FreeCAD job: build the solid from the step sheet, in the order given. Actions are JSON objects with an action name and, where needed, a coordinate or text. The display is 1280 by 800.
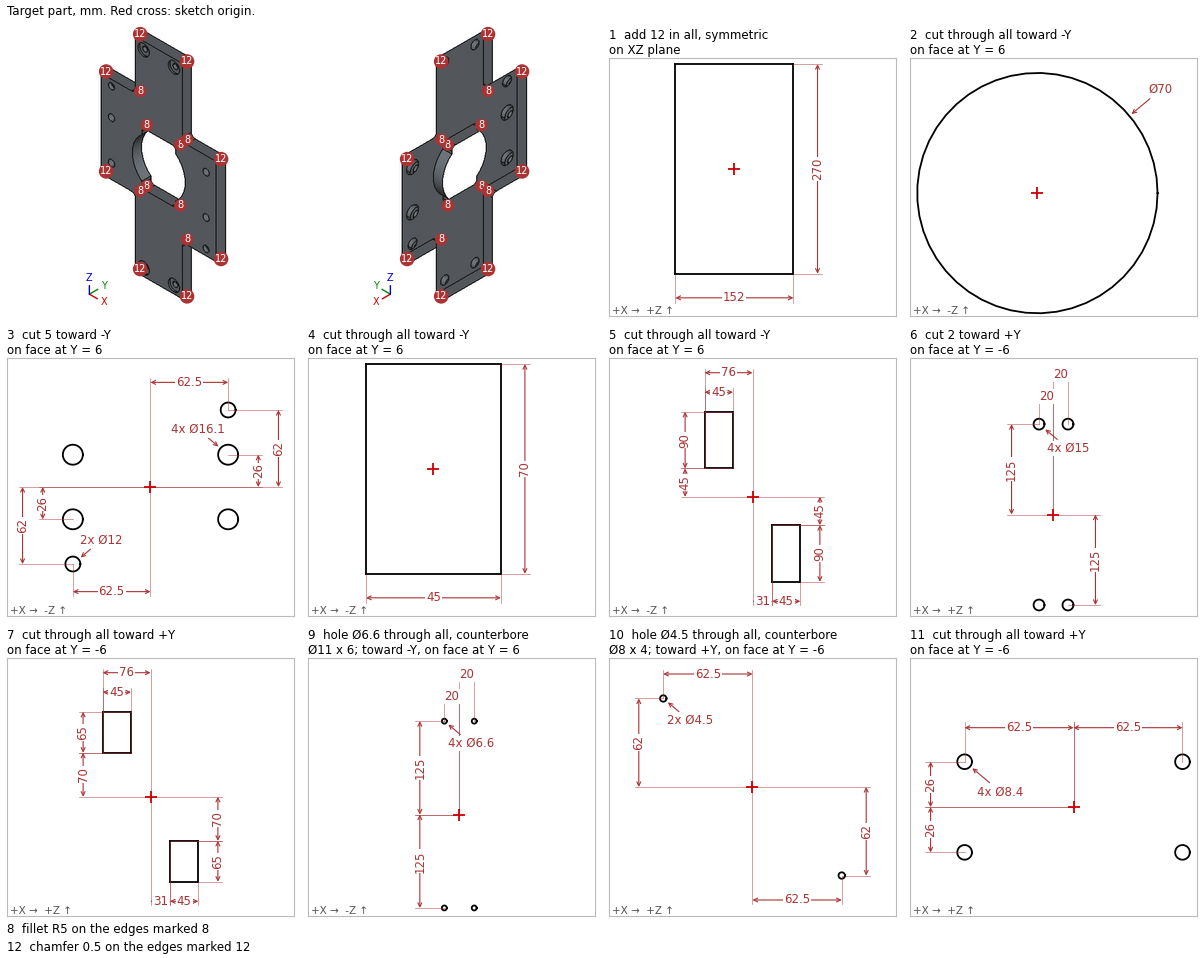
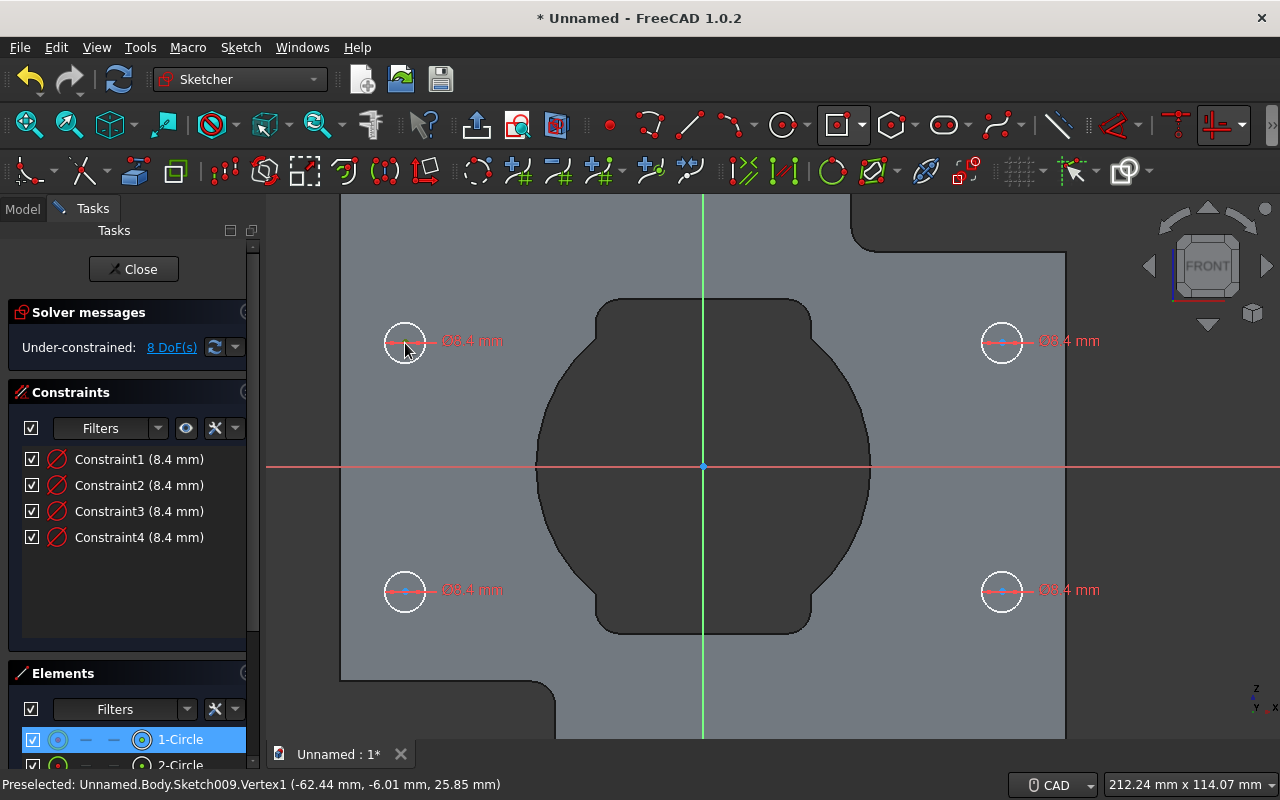
{"action": "left_click", "coordinate": [405, 592]}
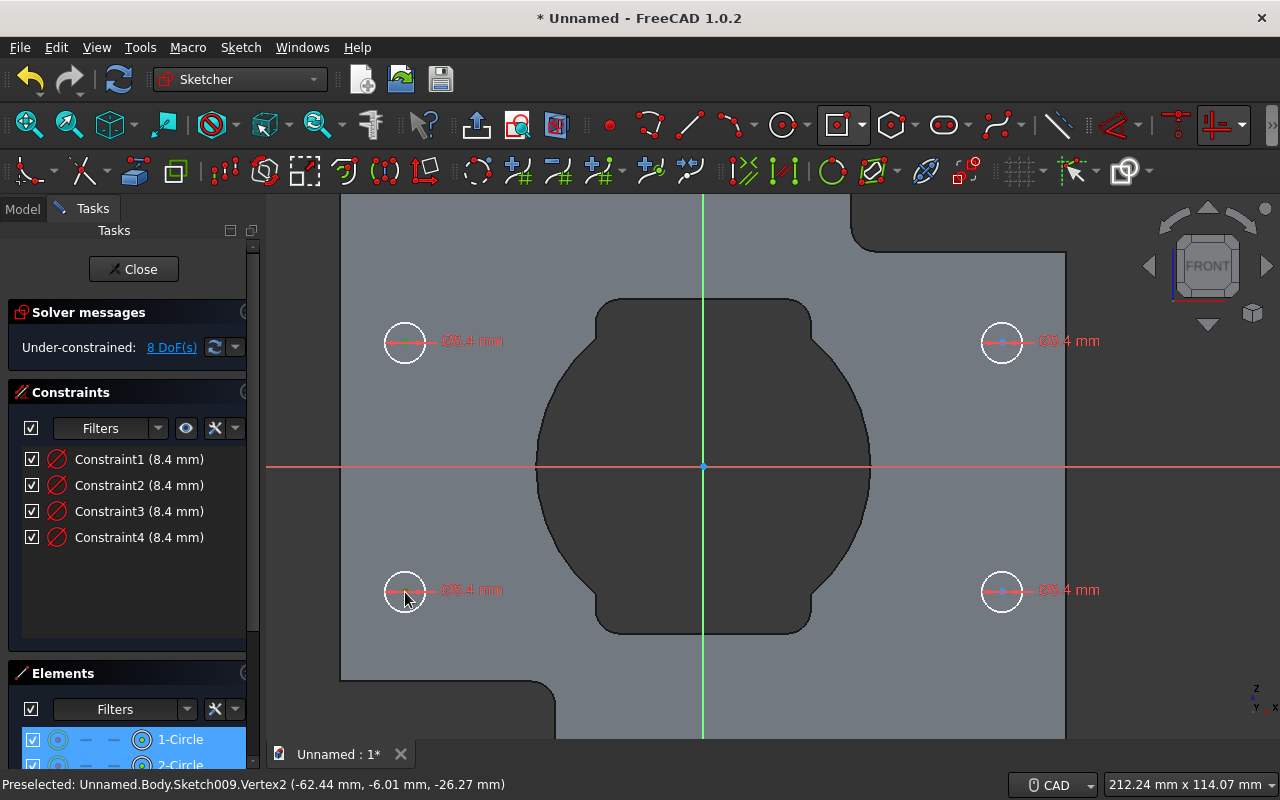
{"action": "key", "text": "v"}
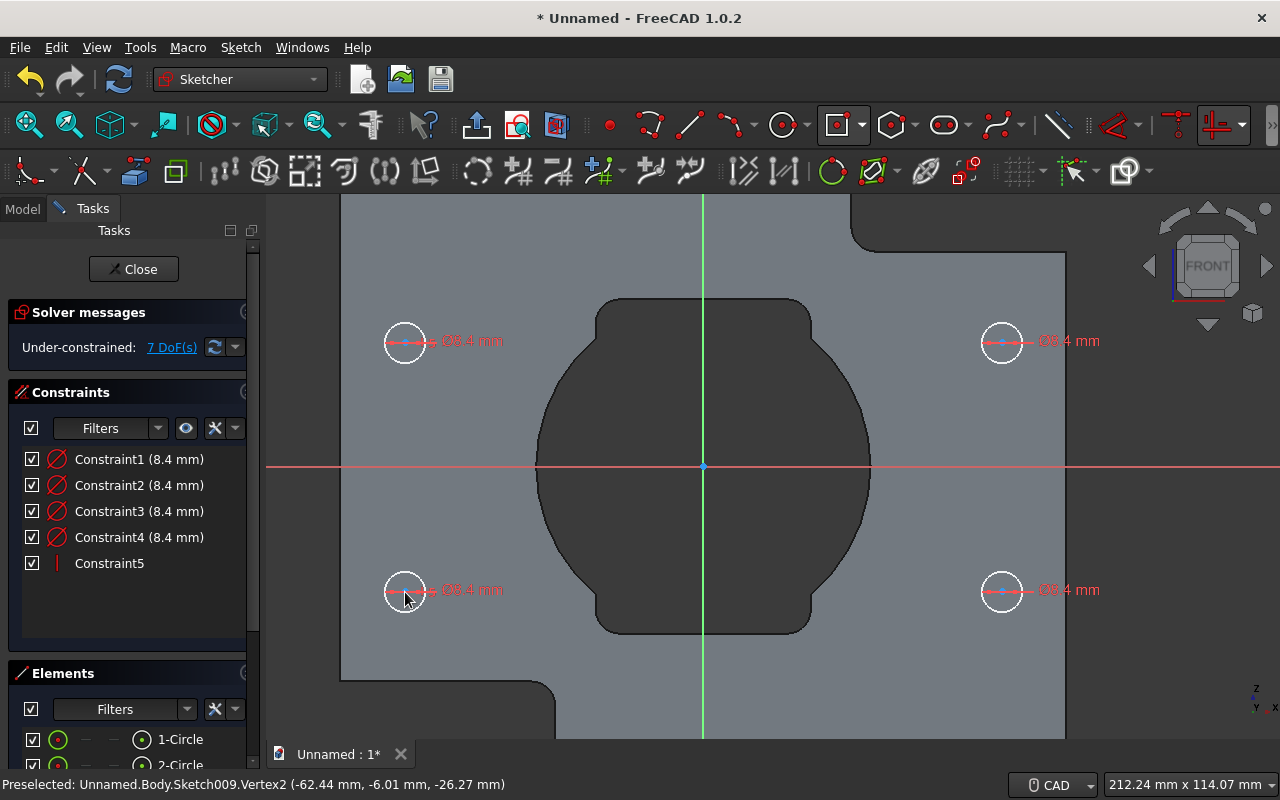
{"action": "left_click", "coordinate": [405, 343]}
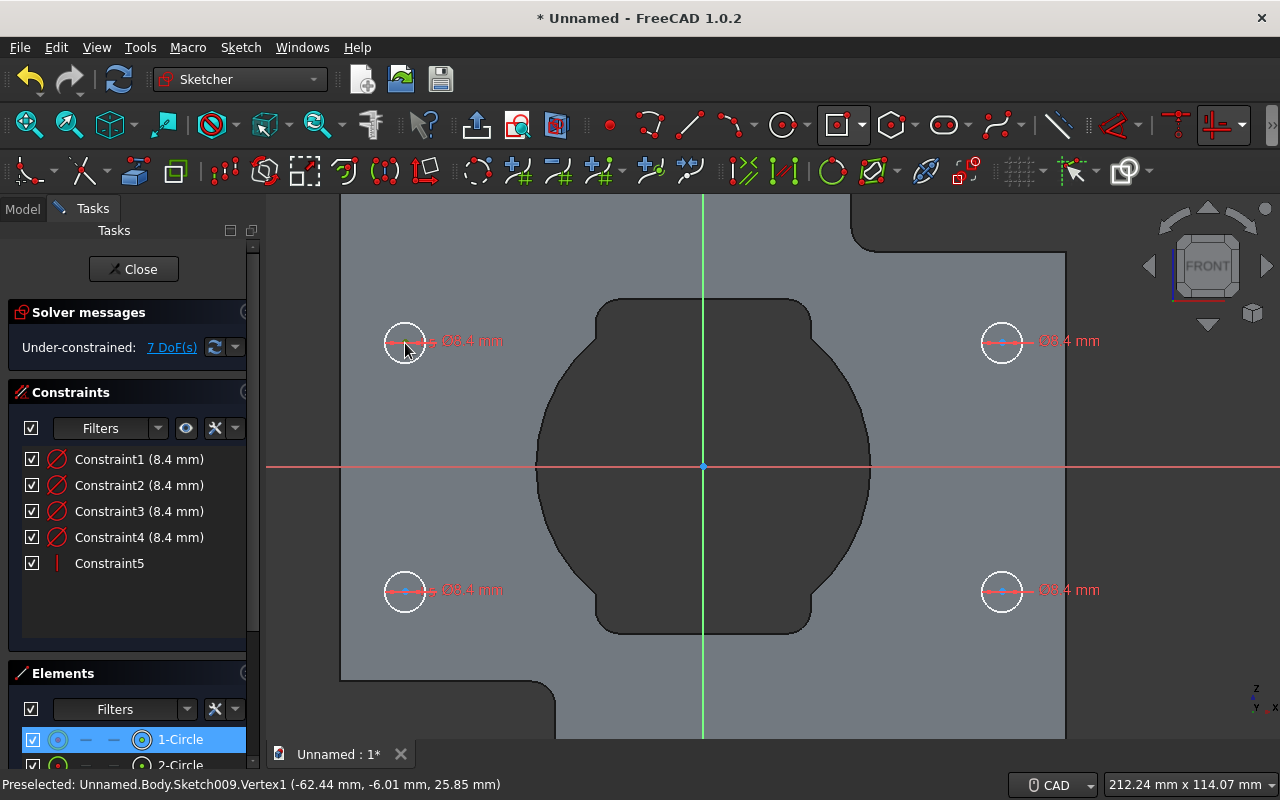
{"action": "left_click", "coordinate": [1002, 343]}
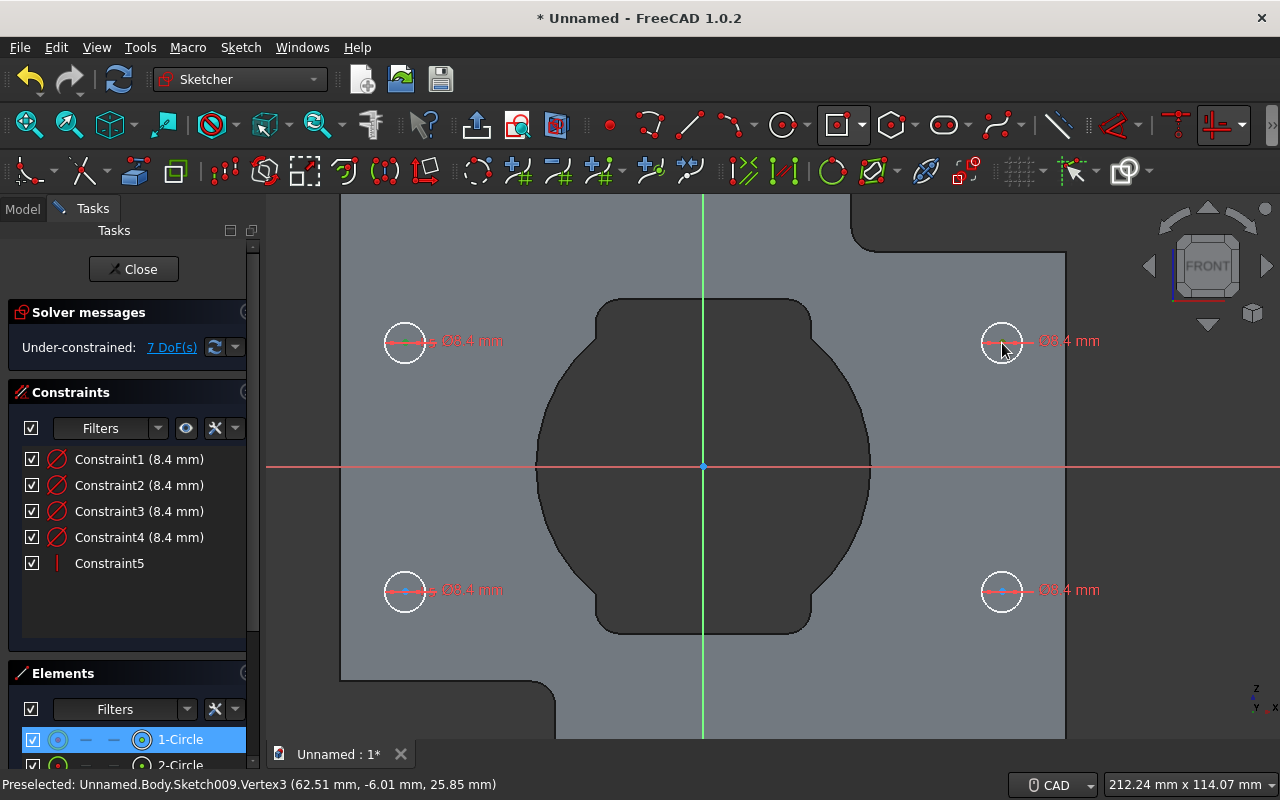
{"action": "left_click", "coordinate": [1244, 126]}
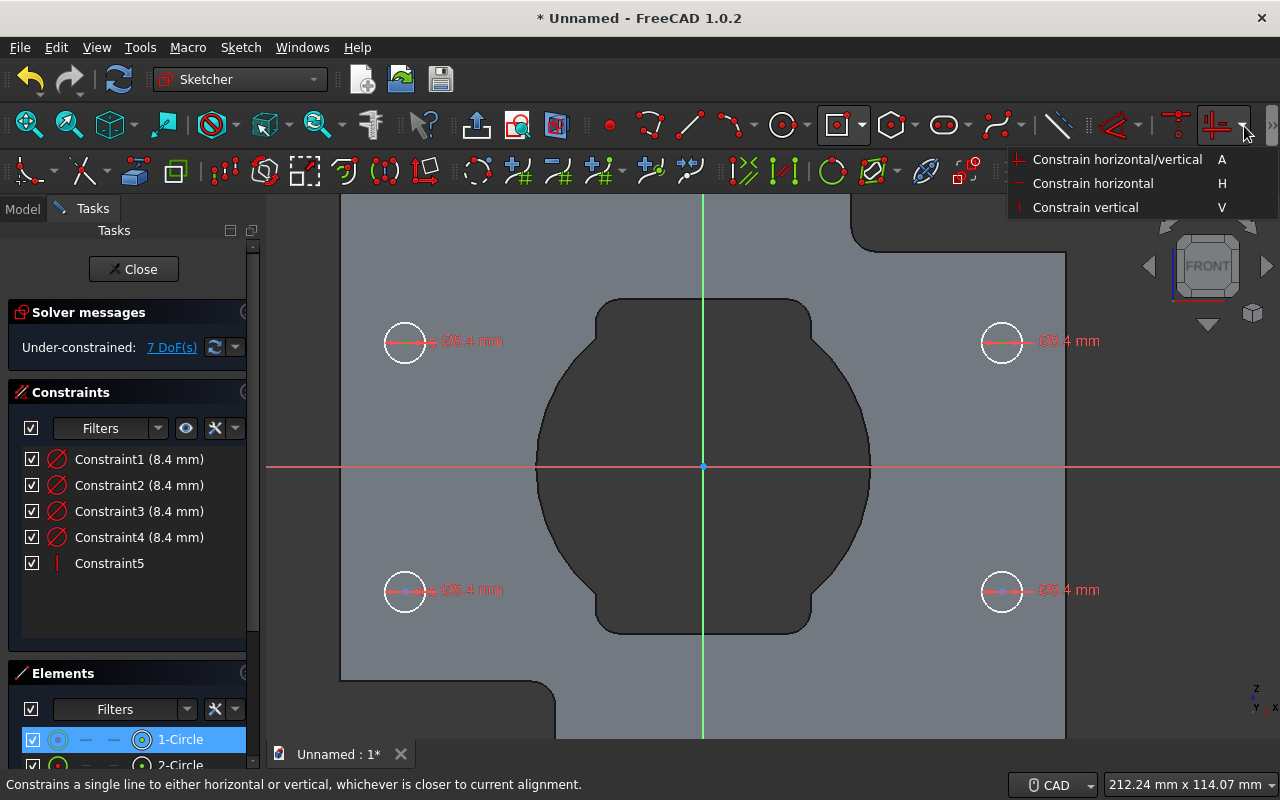
{"action": "left_click", "coordinate": [1143, 183]}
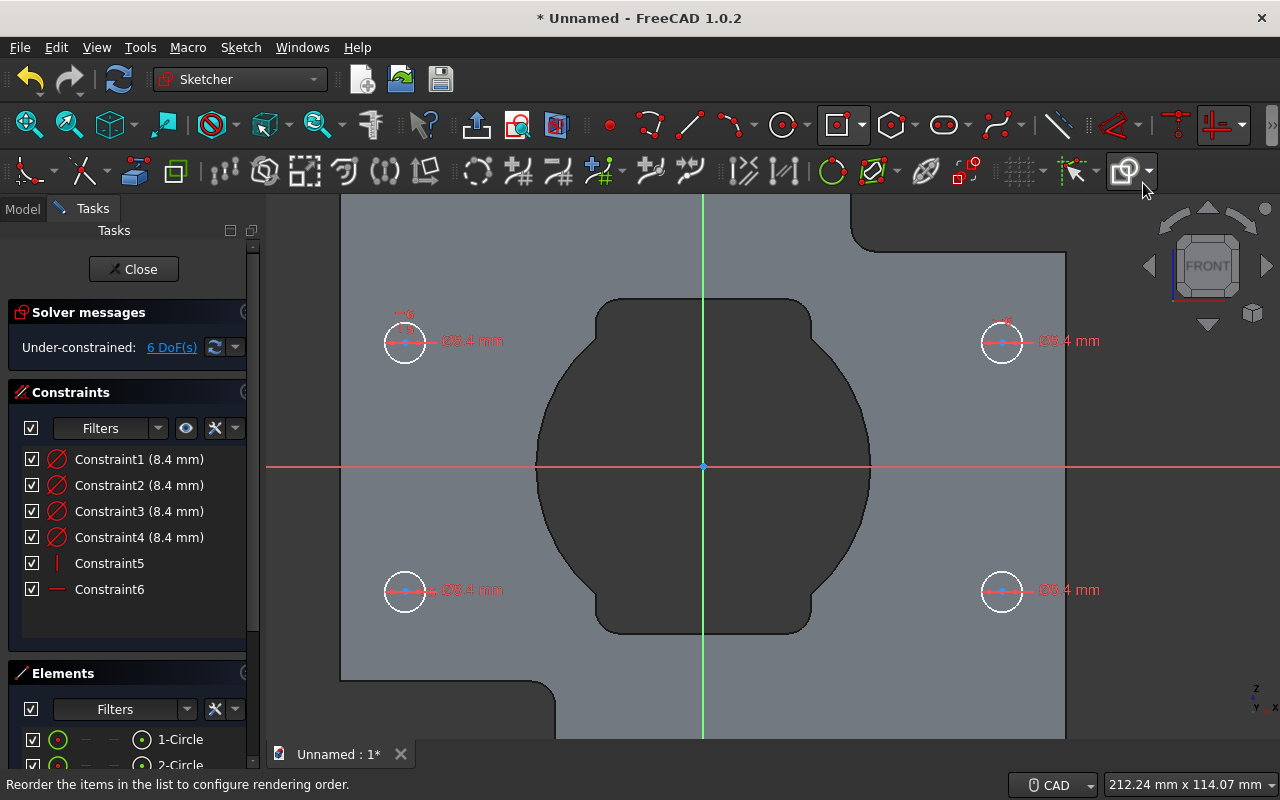
{"action": "left_click", "coordinate": [1002, 343]}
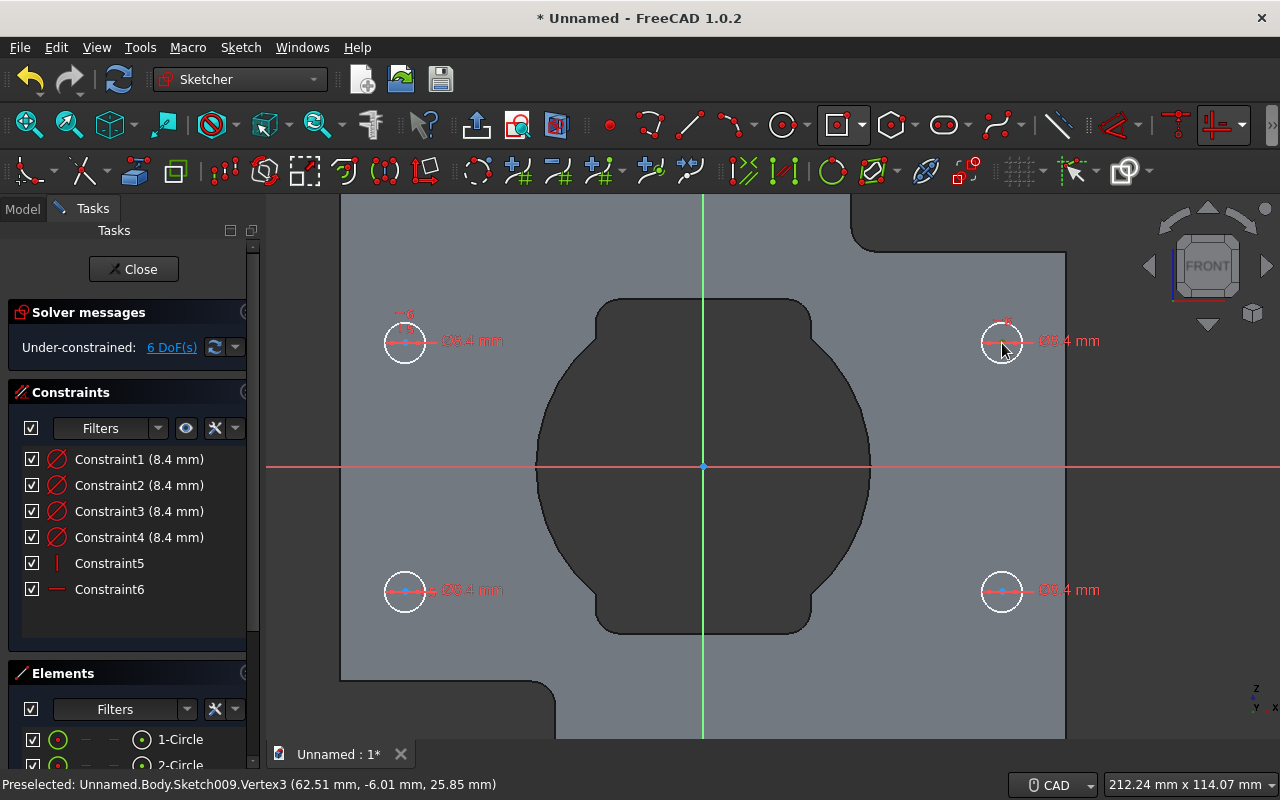
{"action": "left_click", "coordinate": [1002, 592]}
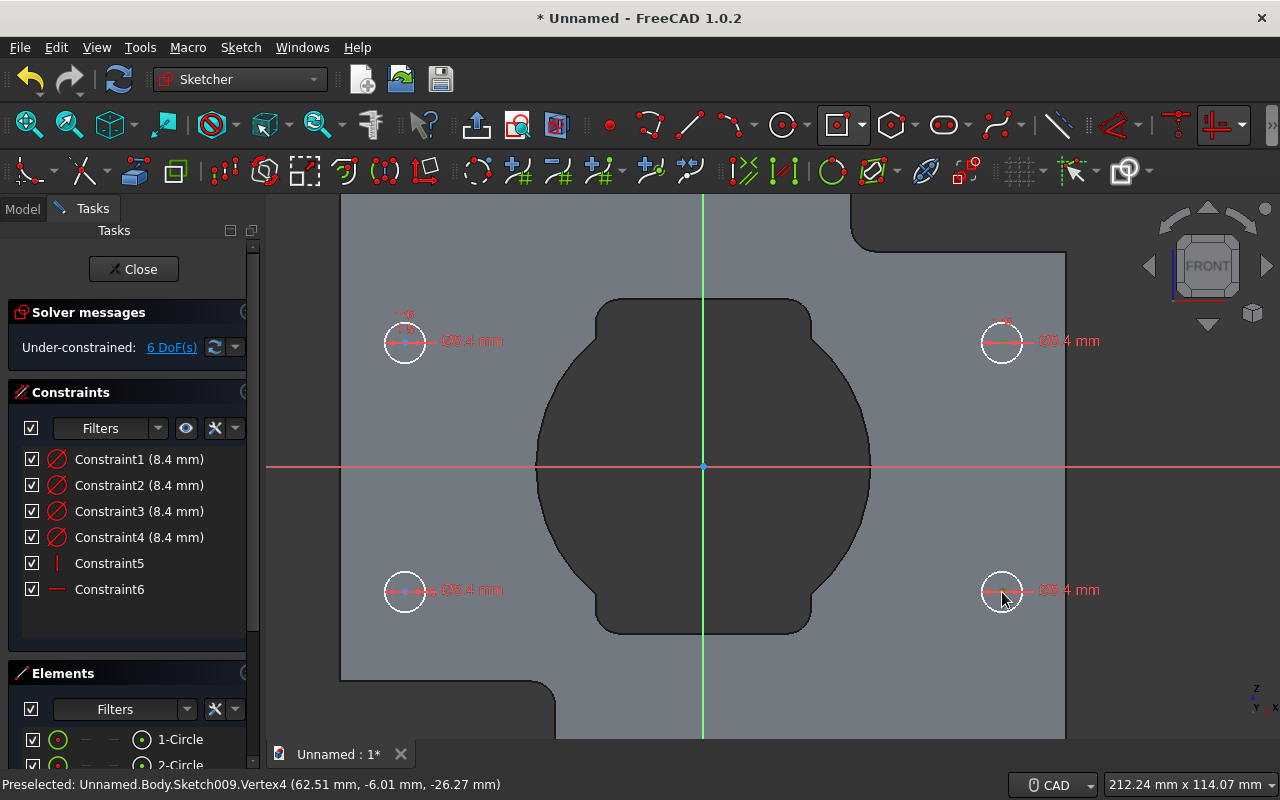
{"action": "key", "text": "v"}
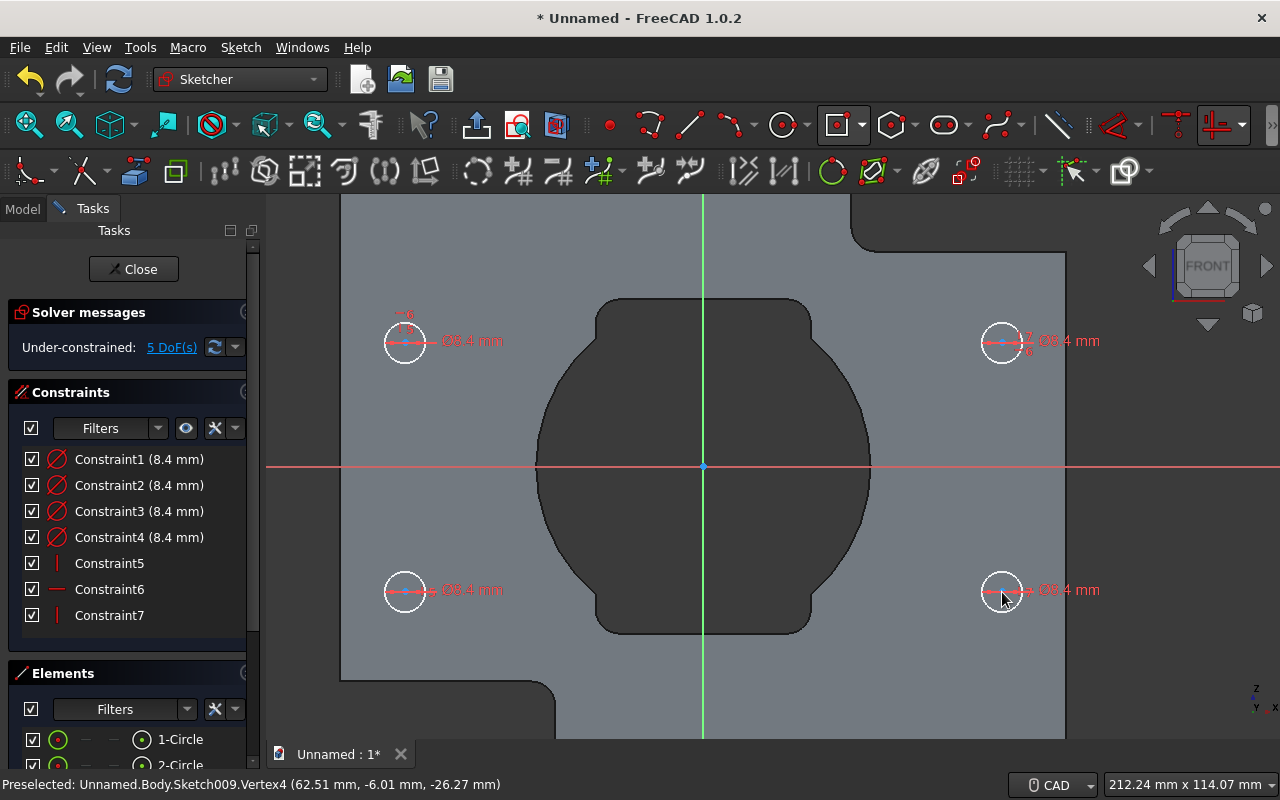
{"action": "left_click", "coordinate": [405, 592]}